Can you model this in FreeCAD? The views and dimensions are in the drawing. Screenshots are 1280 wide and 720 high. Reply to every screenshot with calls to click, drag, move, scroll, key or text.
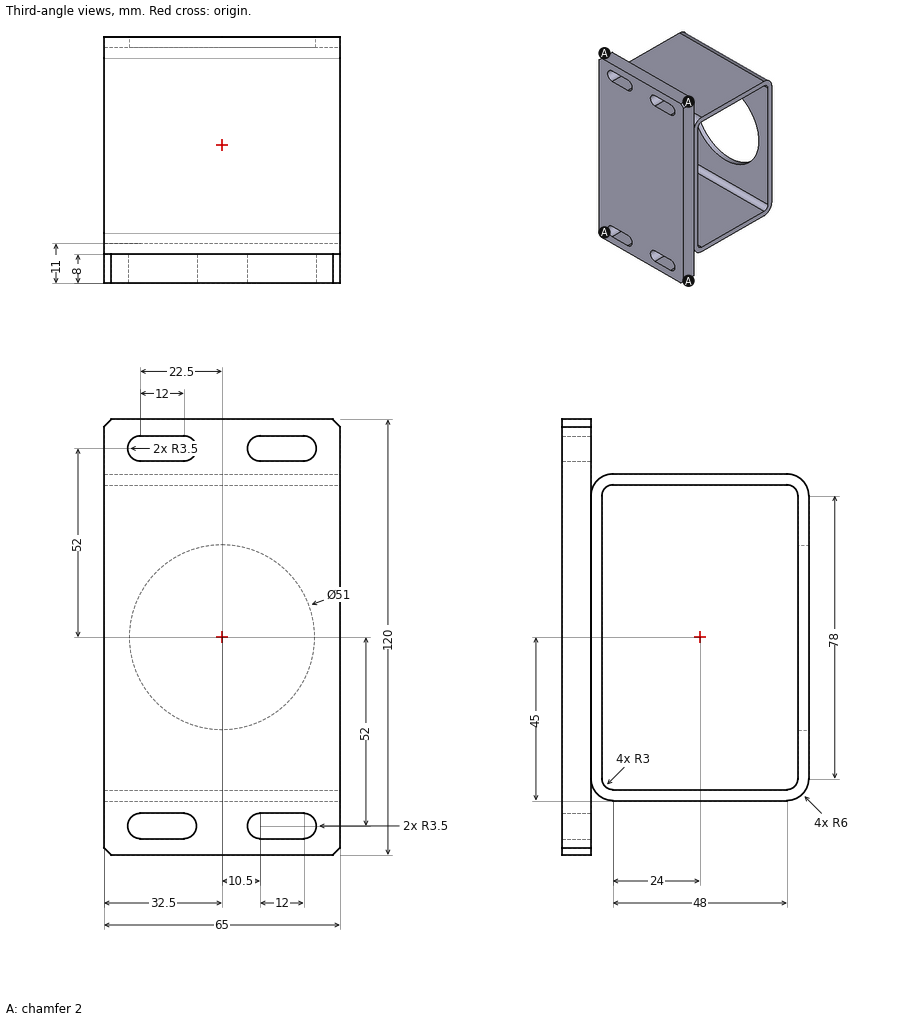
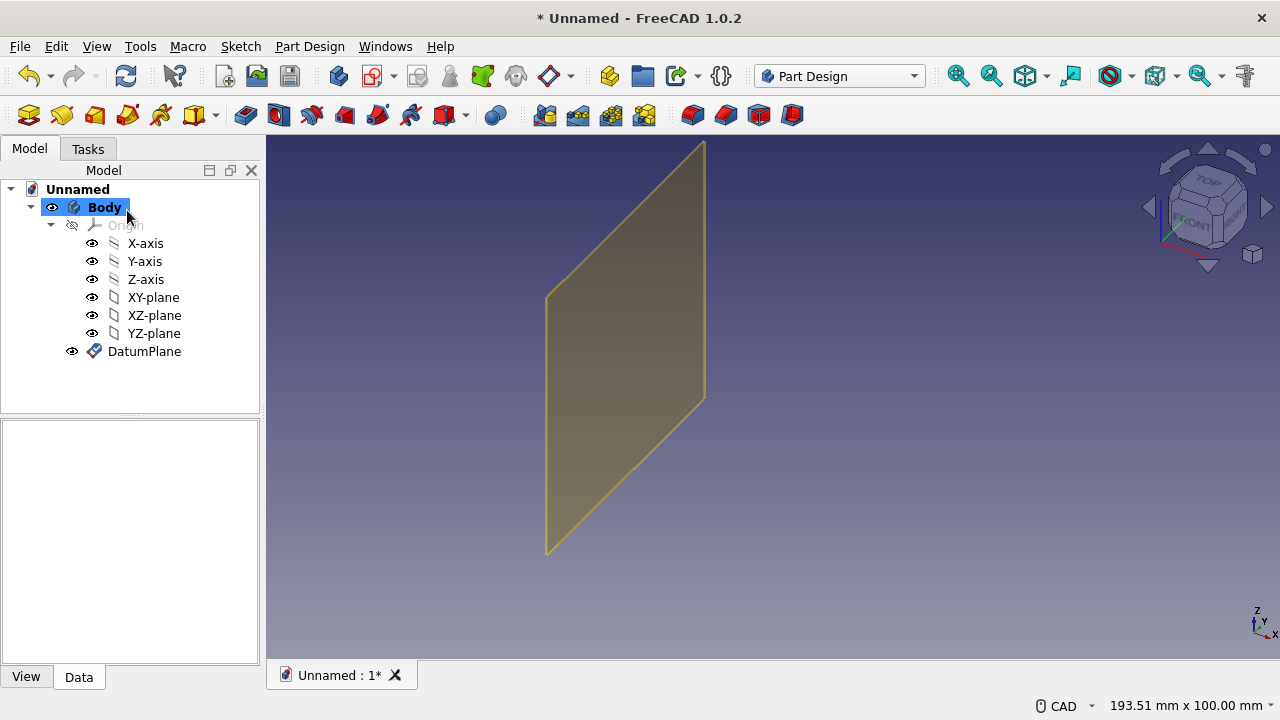
click(117, 351)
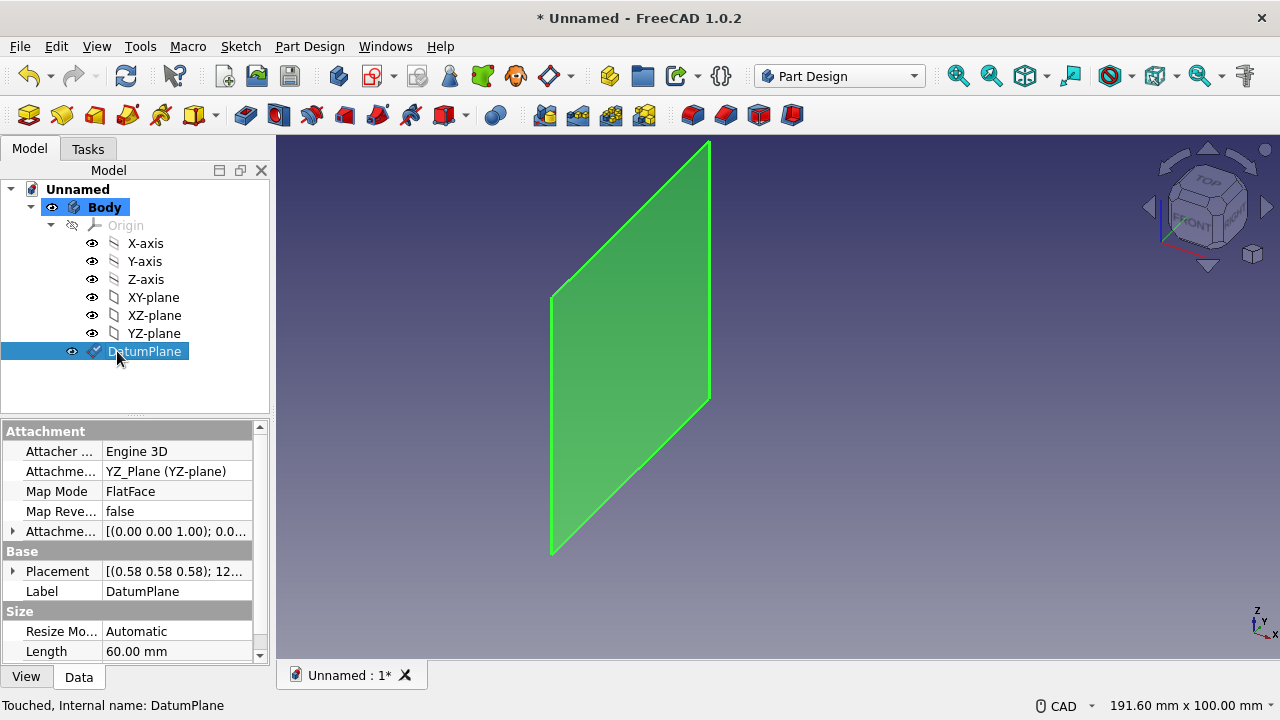
click(372, 76)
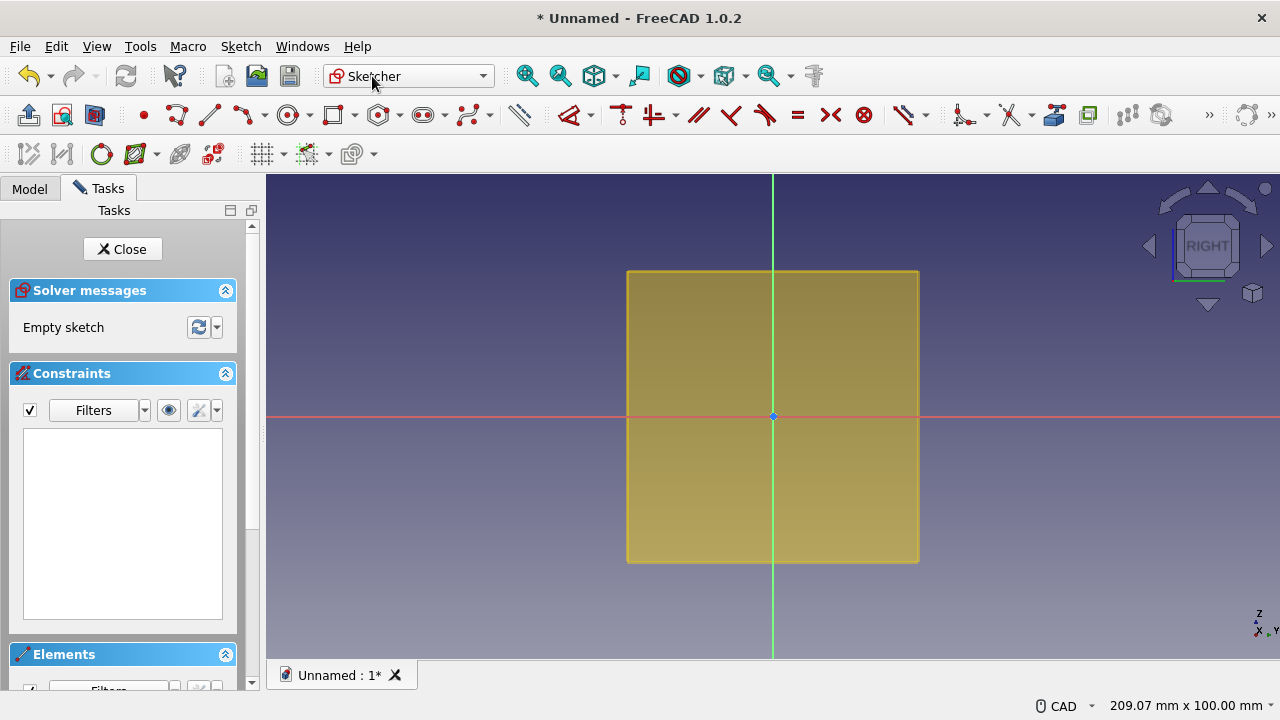
scroll(565, 416, down, 2)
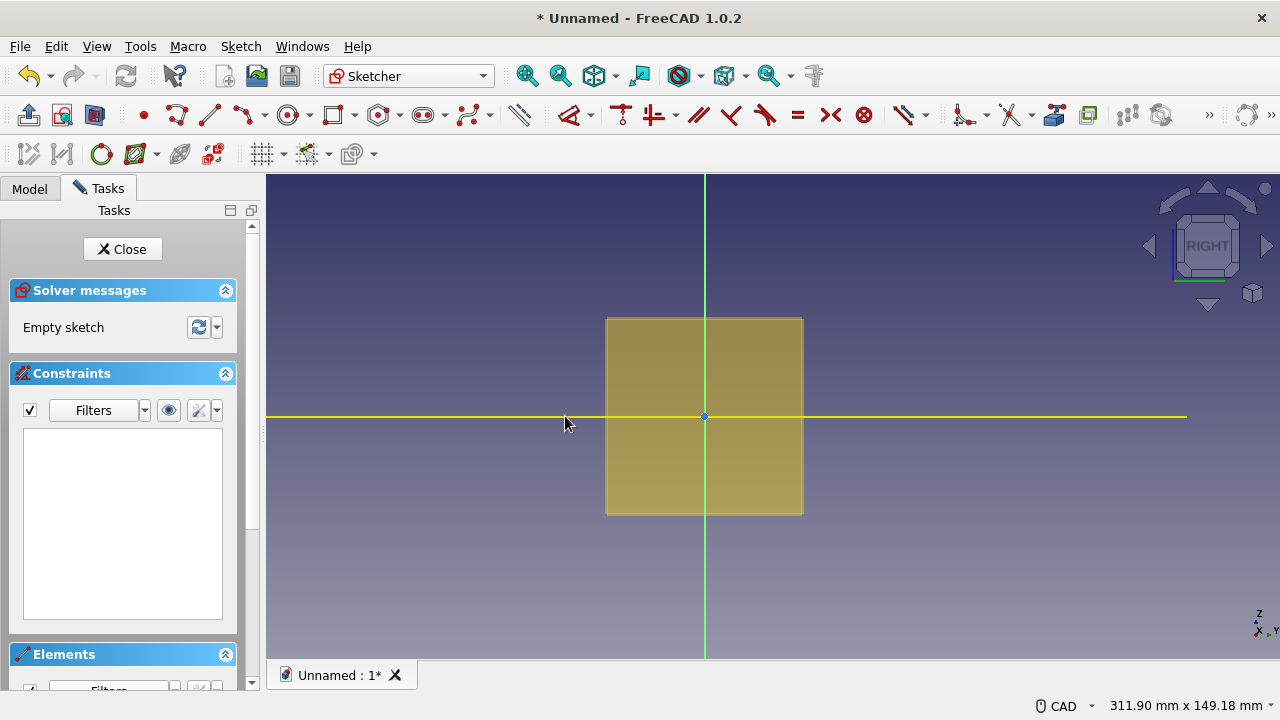
click(210, 116)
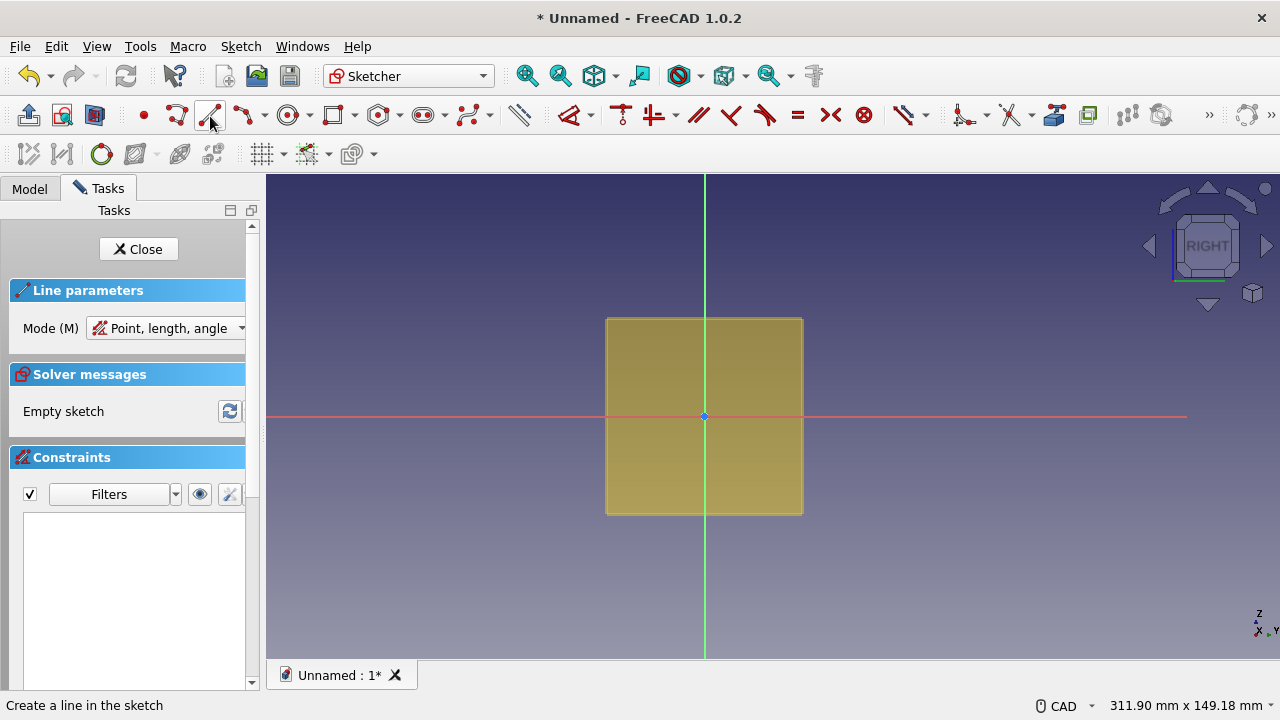
click(626, 563)
click(783, 563)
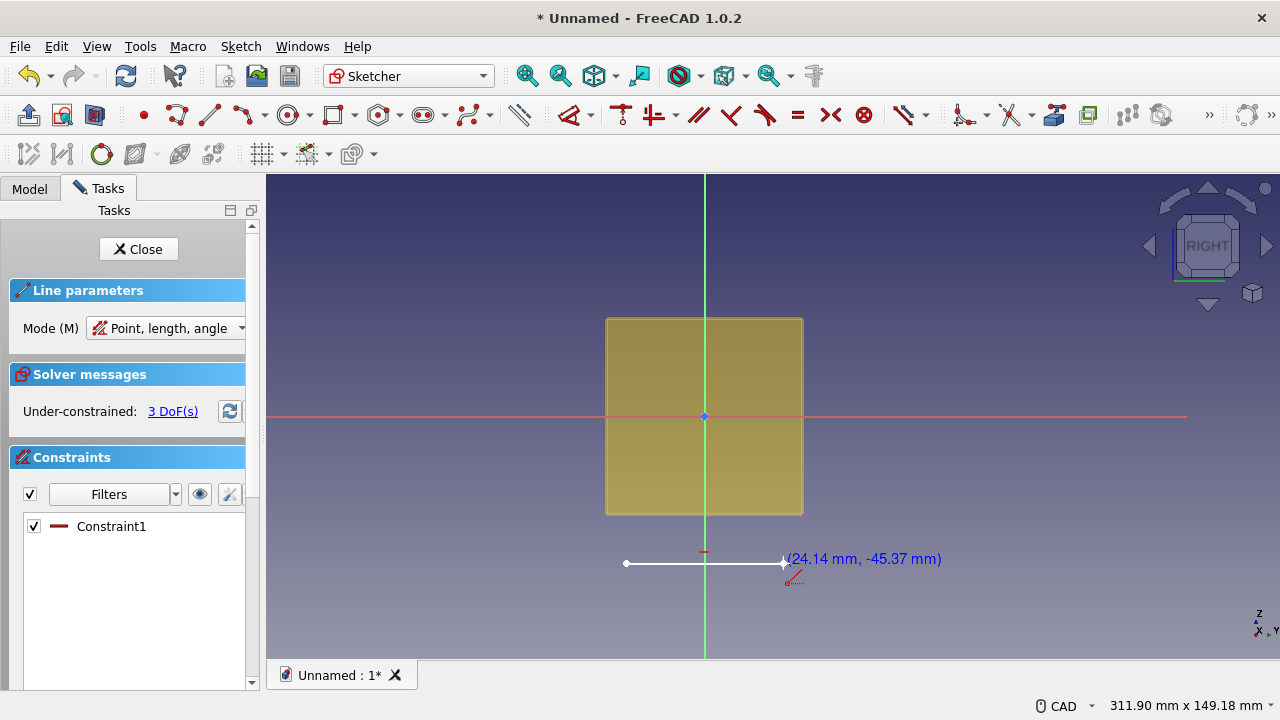
click(802, 543)
click(802, 290)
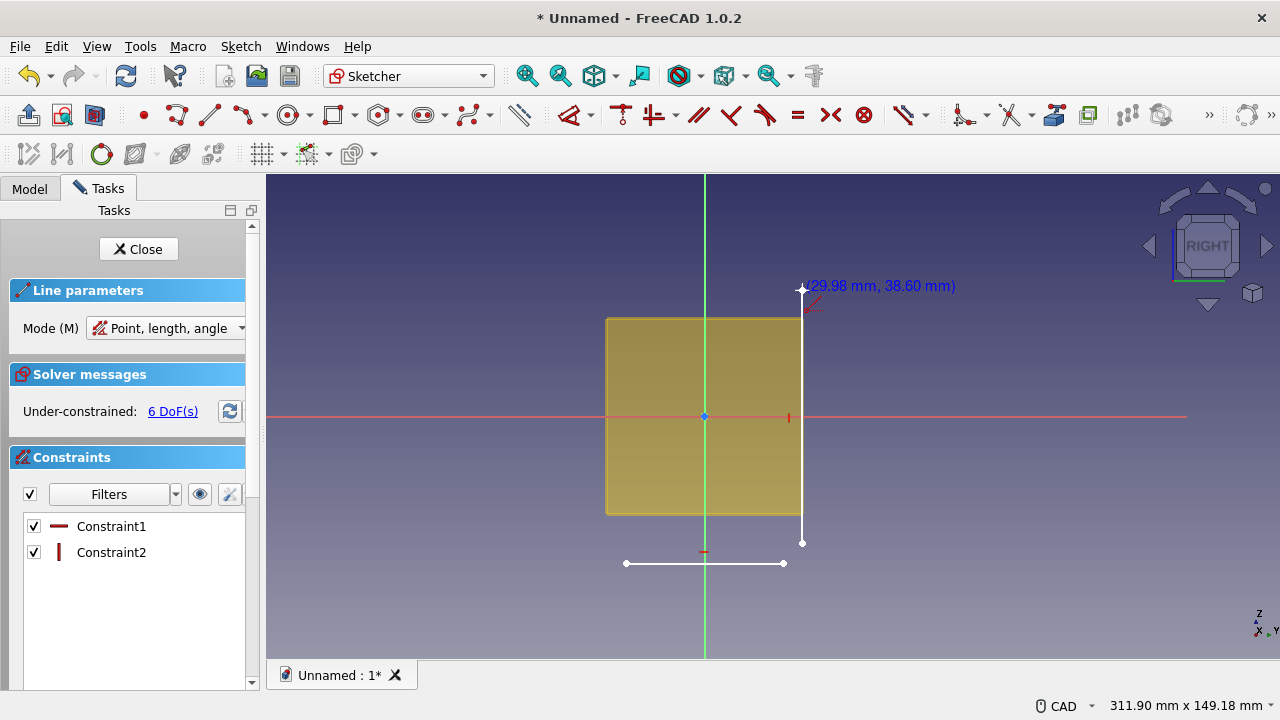
click(783, 270)
click(626, 270)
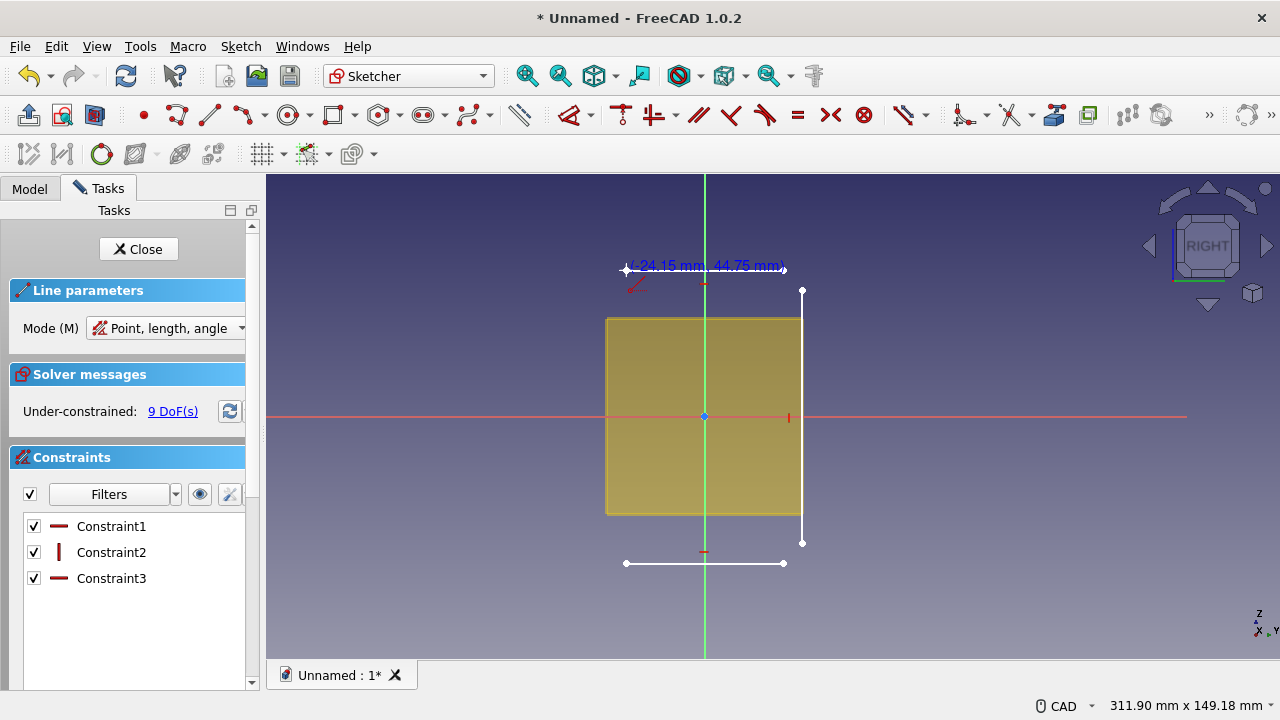
click(607, 290)
click(607, 543)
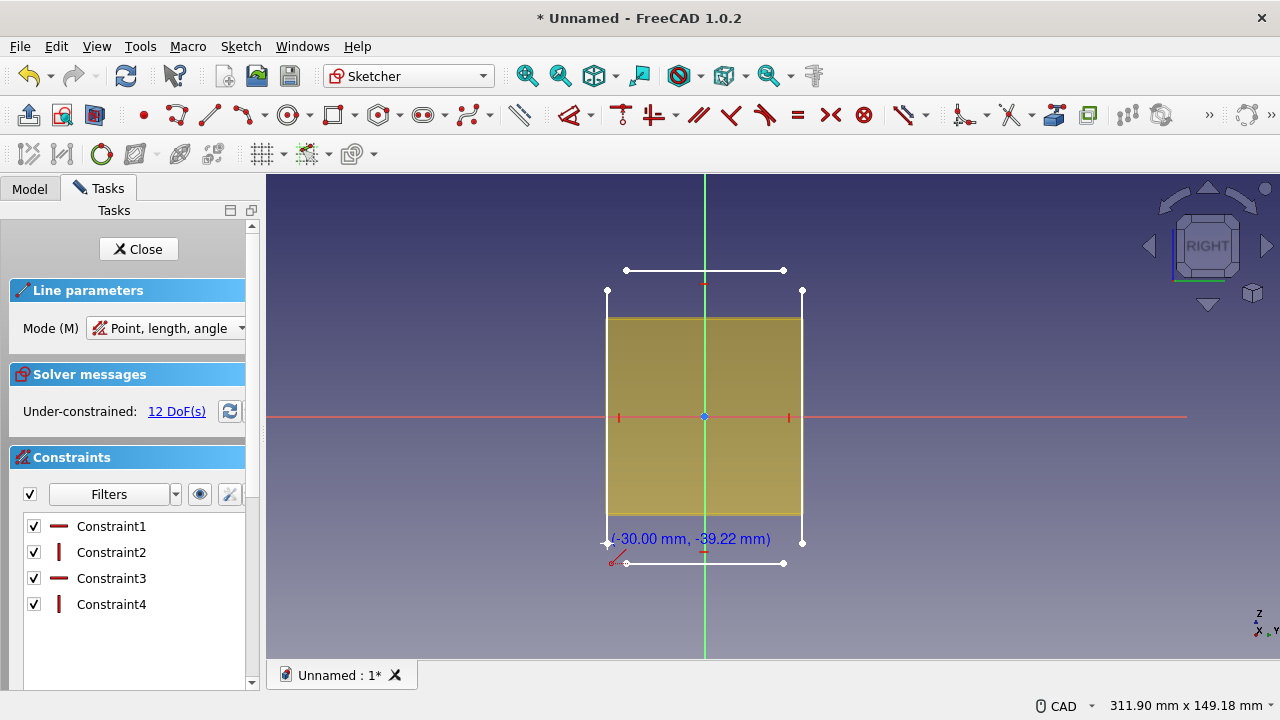
click(242, 116)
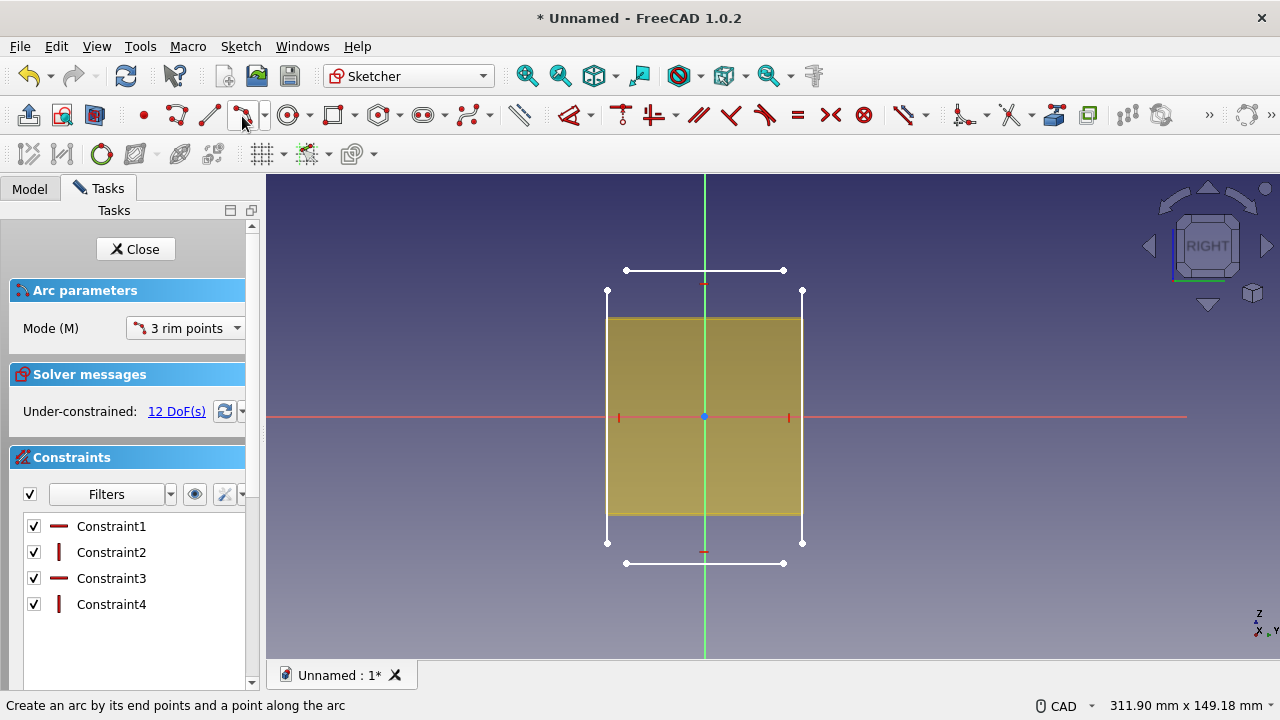
click(783, 564)
click(802, 544)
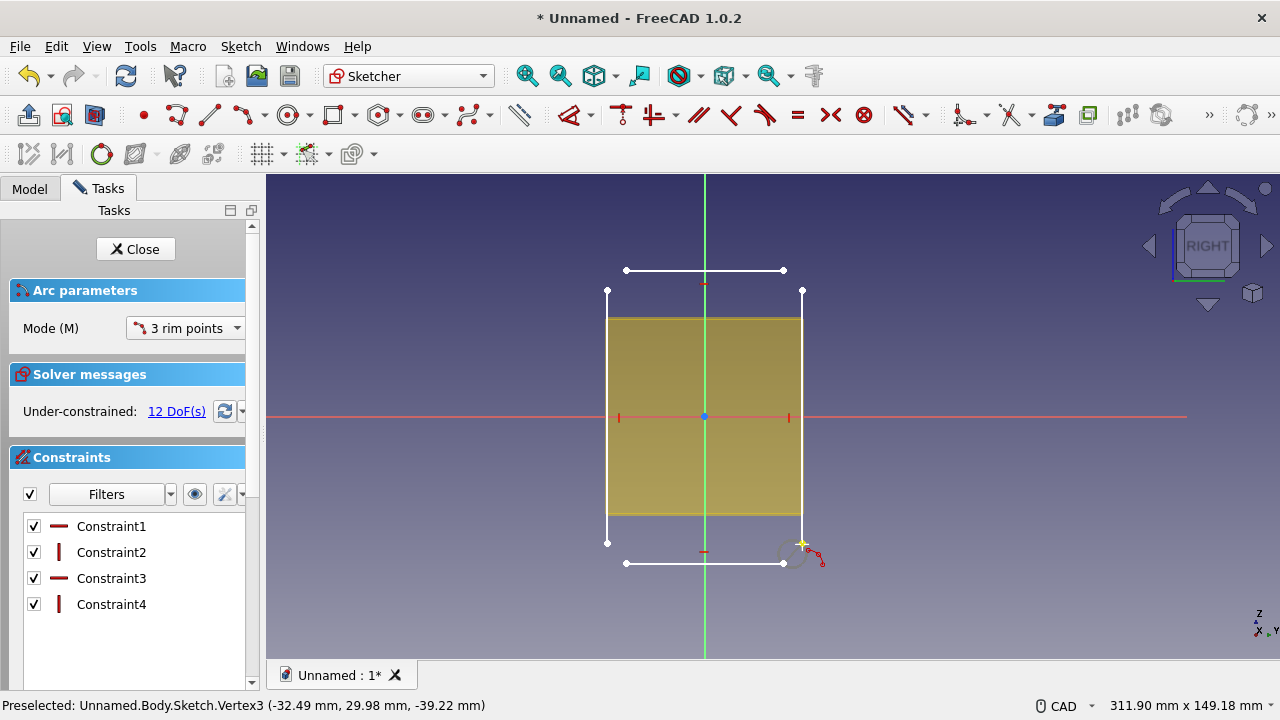
scroll(796, 557, up, 6)